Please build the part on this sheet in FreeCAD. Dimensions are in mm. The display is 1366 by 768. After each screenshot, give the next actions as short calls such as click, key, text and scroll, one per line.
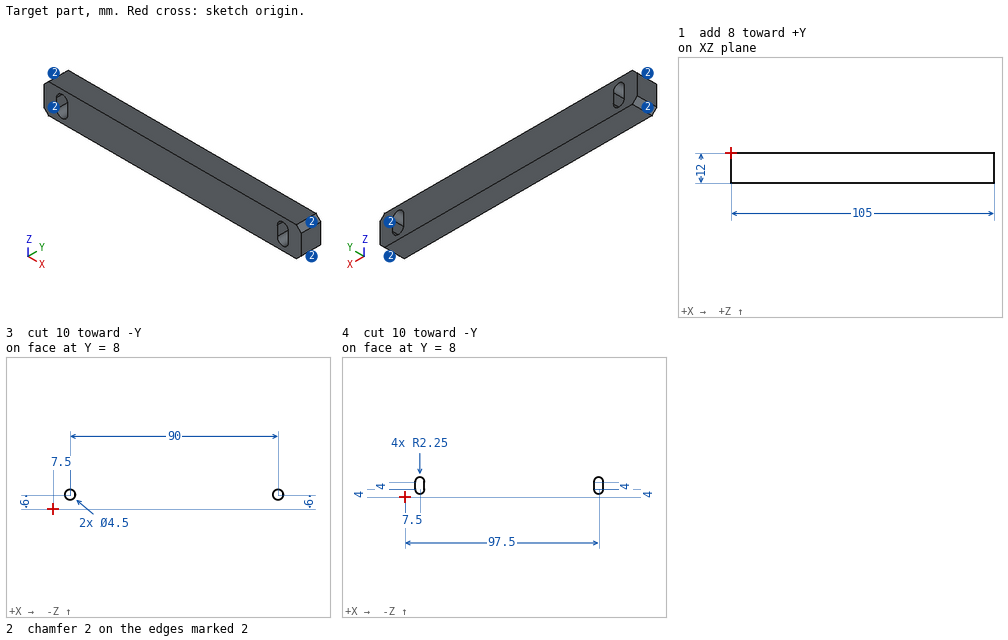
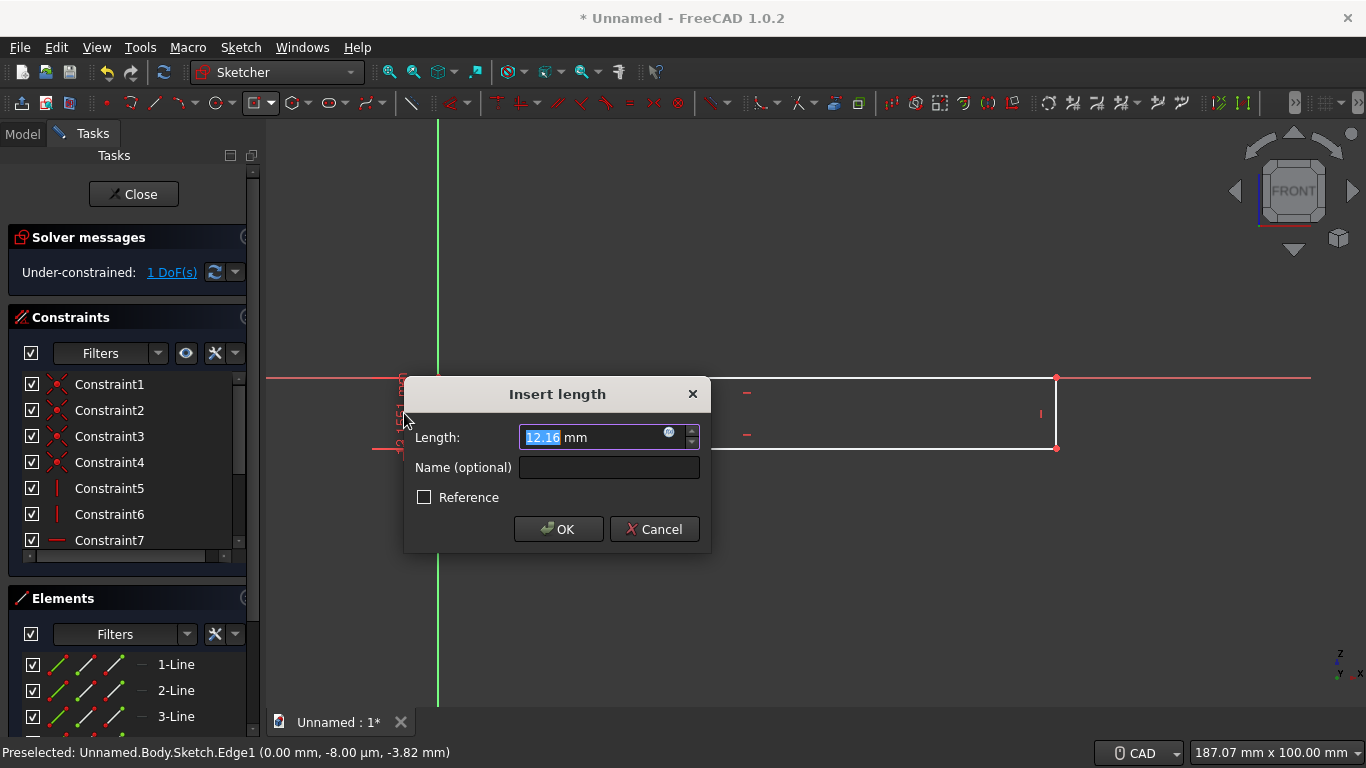
text(12)
key(Return)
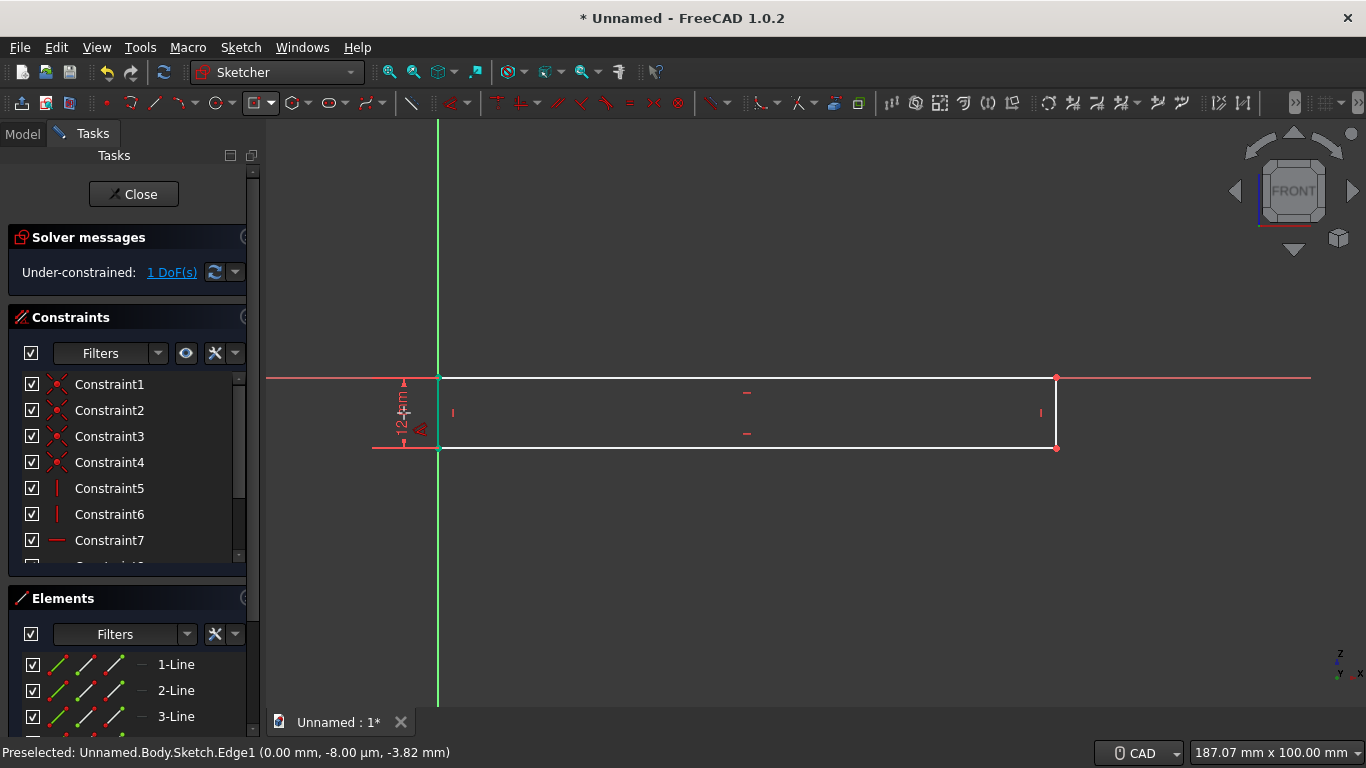
click(624, 448)
click(747, 482)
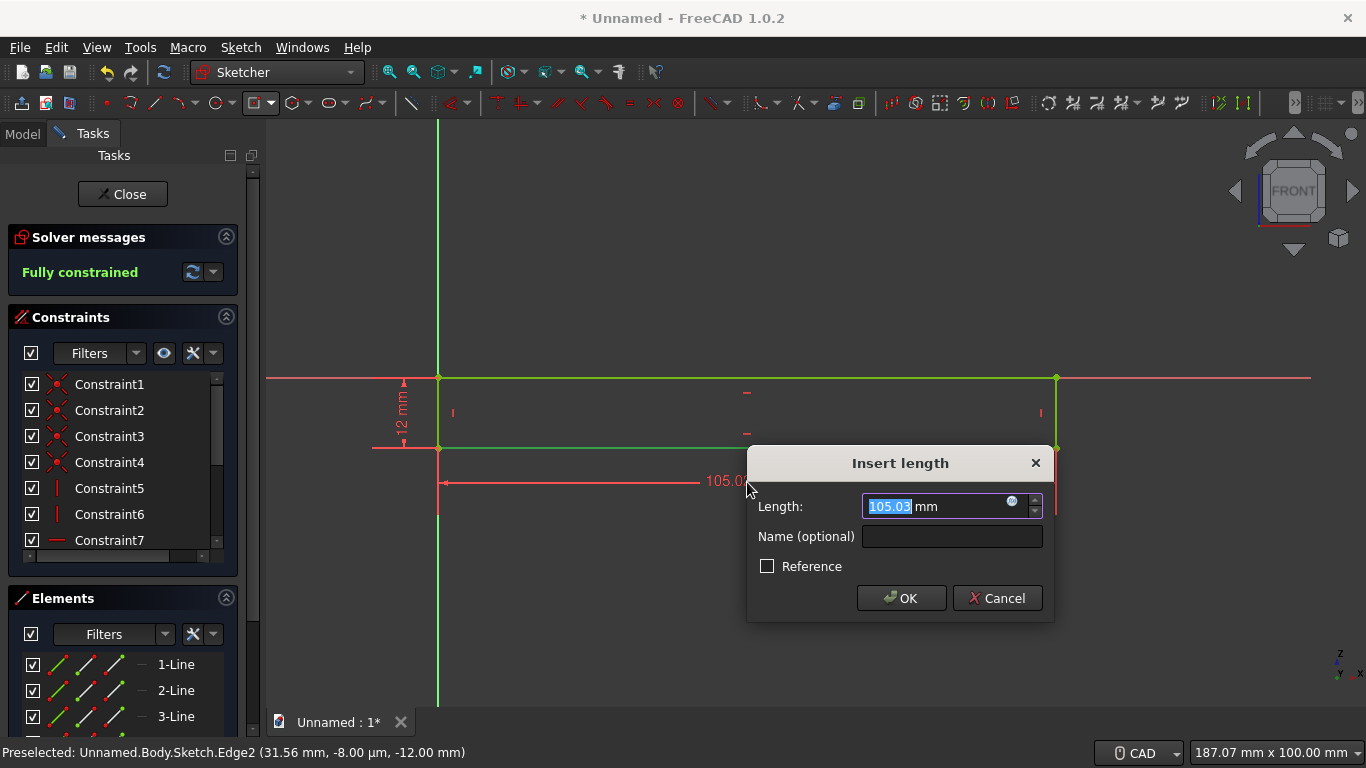
text(105)
key(Return)
key(Escape)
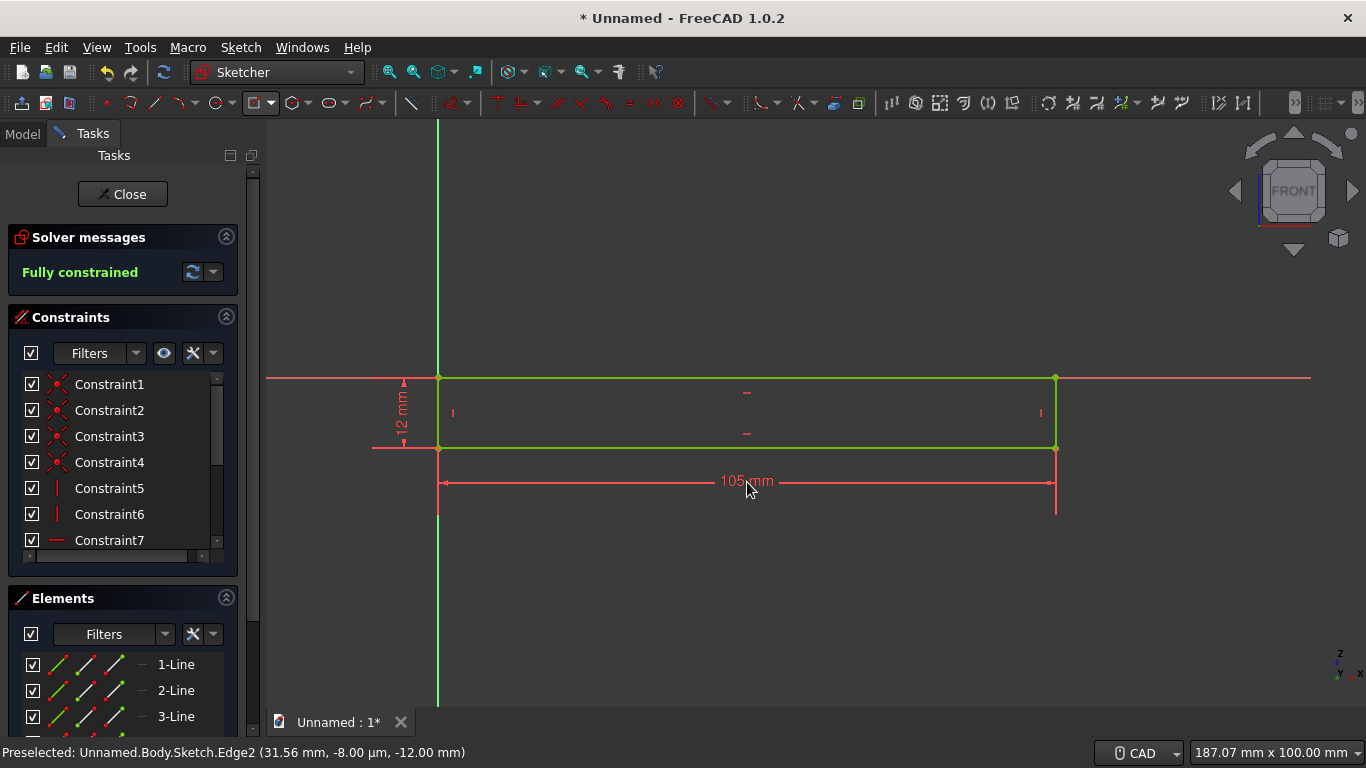
click(123, 194)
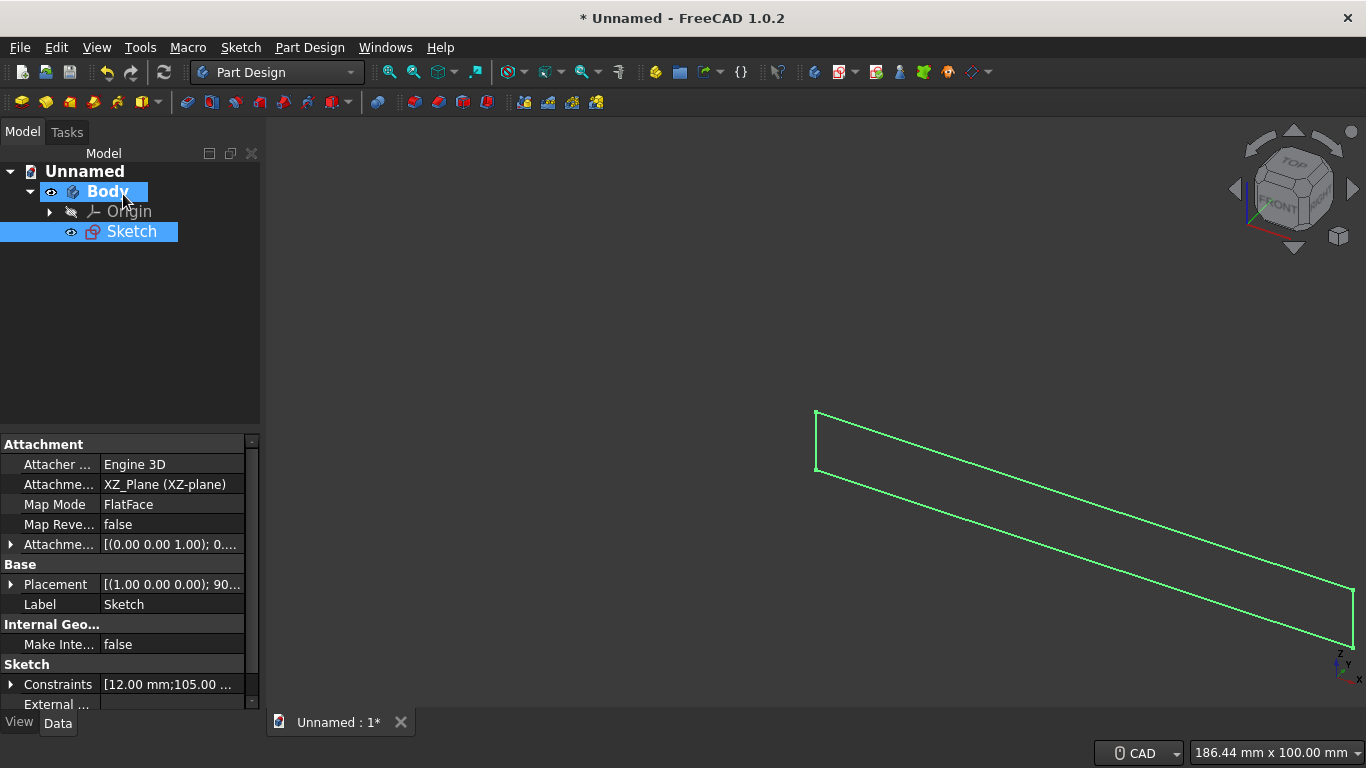
click(22, 102)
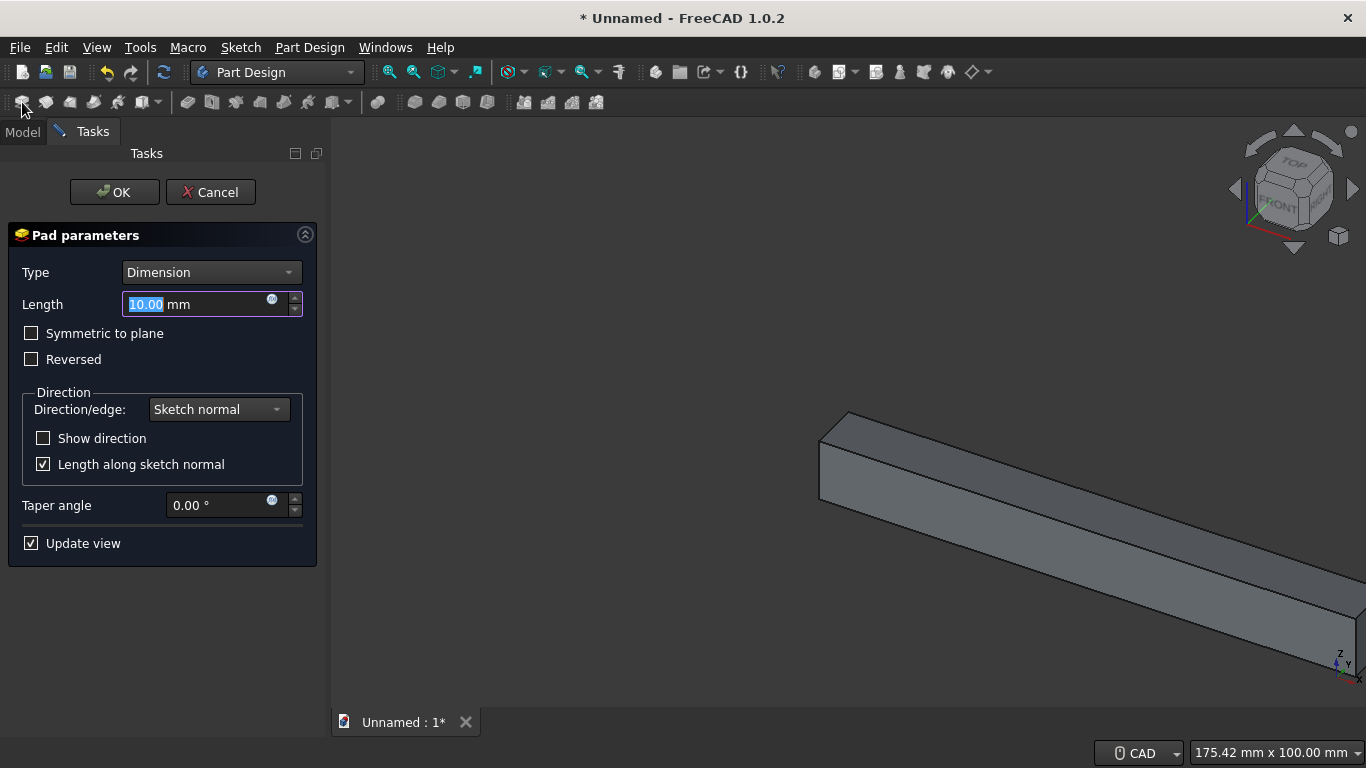
text(8)
key(Tab)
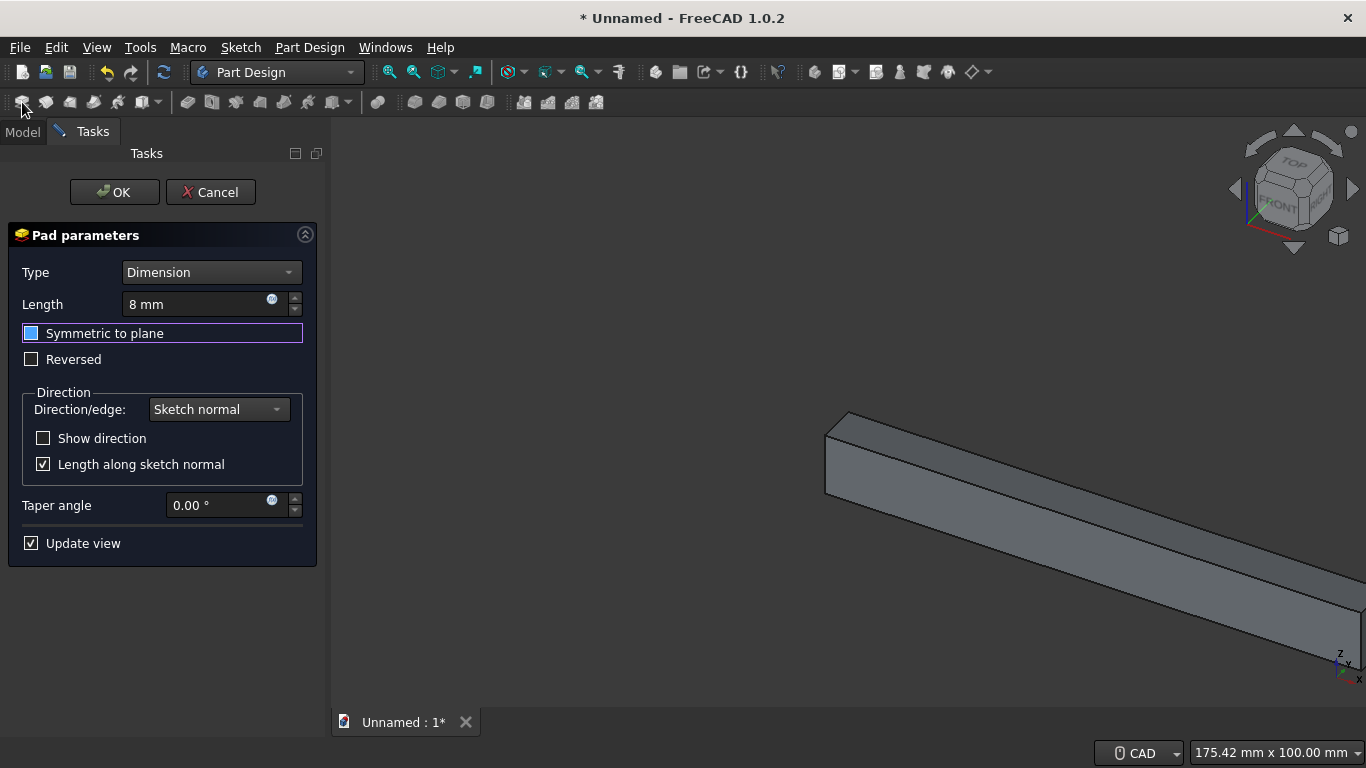
click(30, 359)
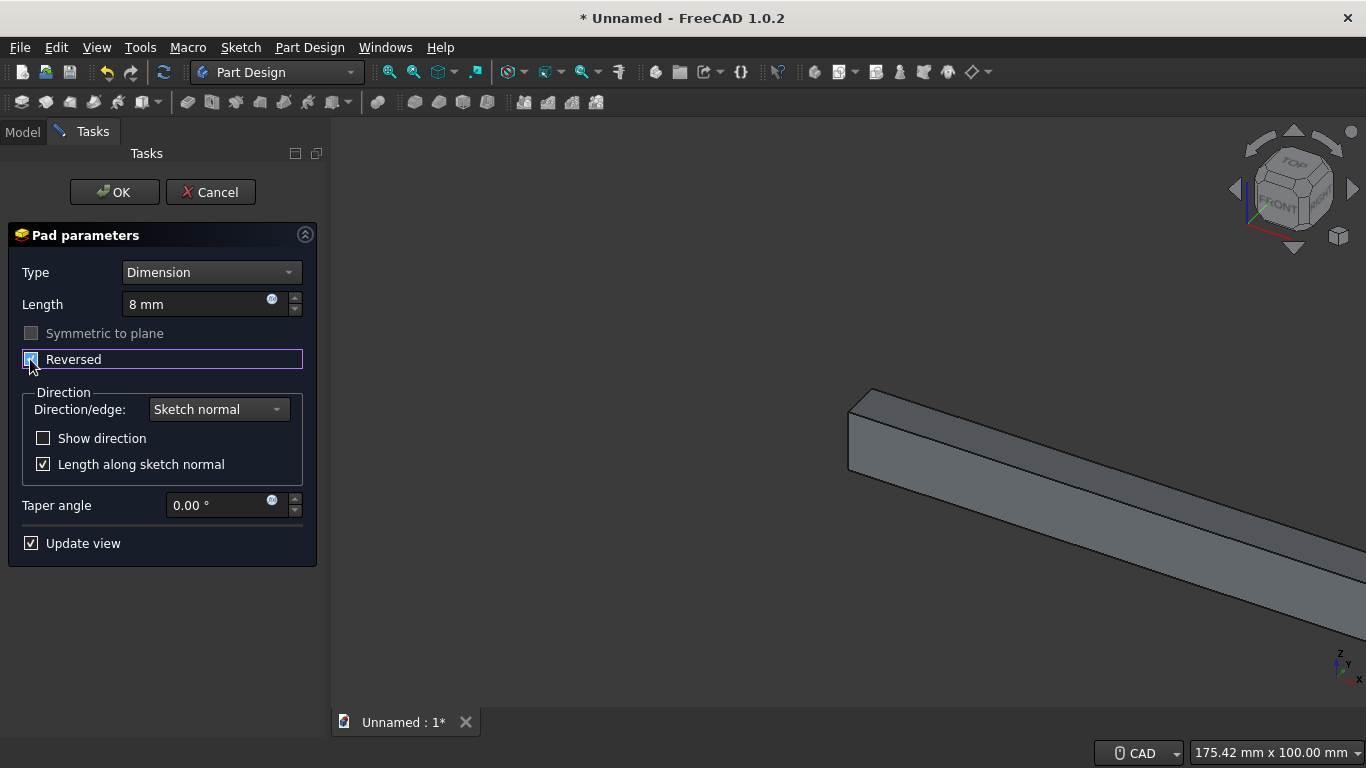
click(115, 192)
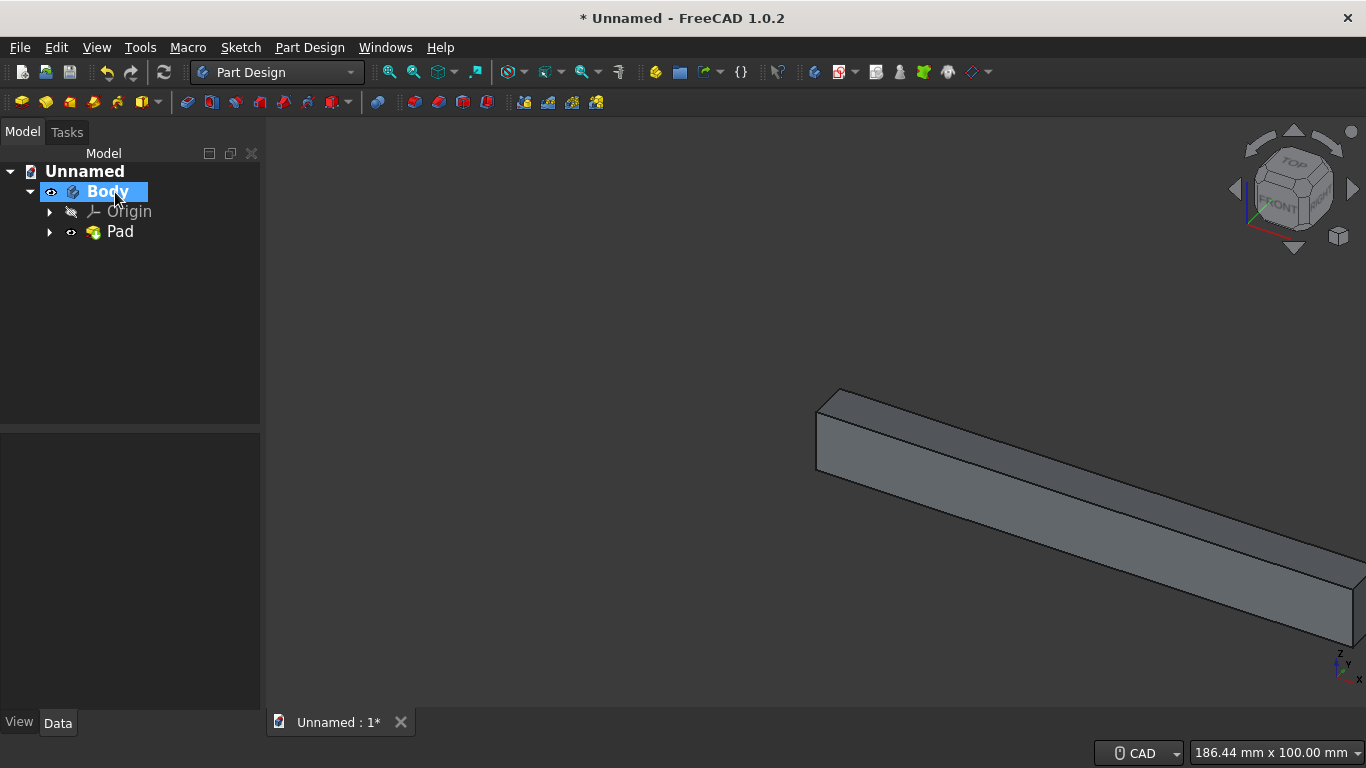
click(390, 72)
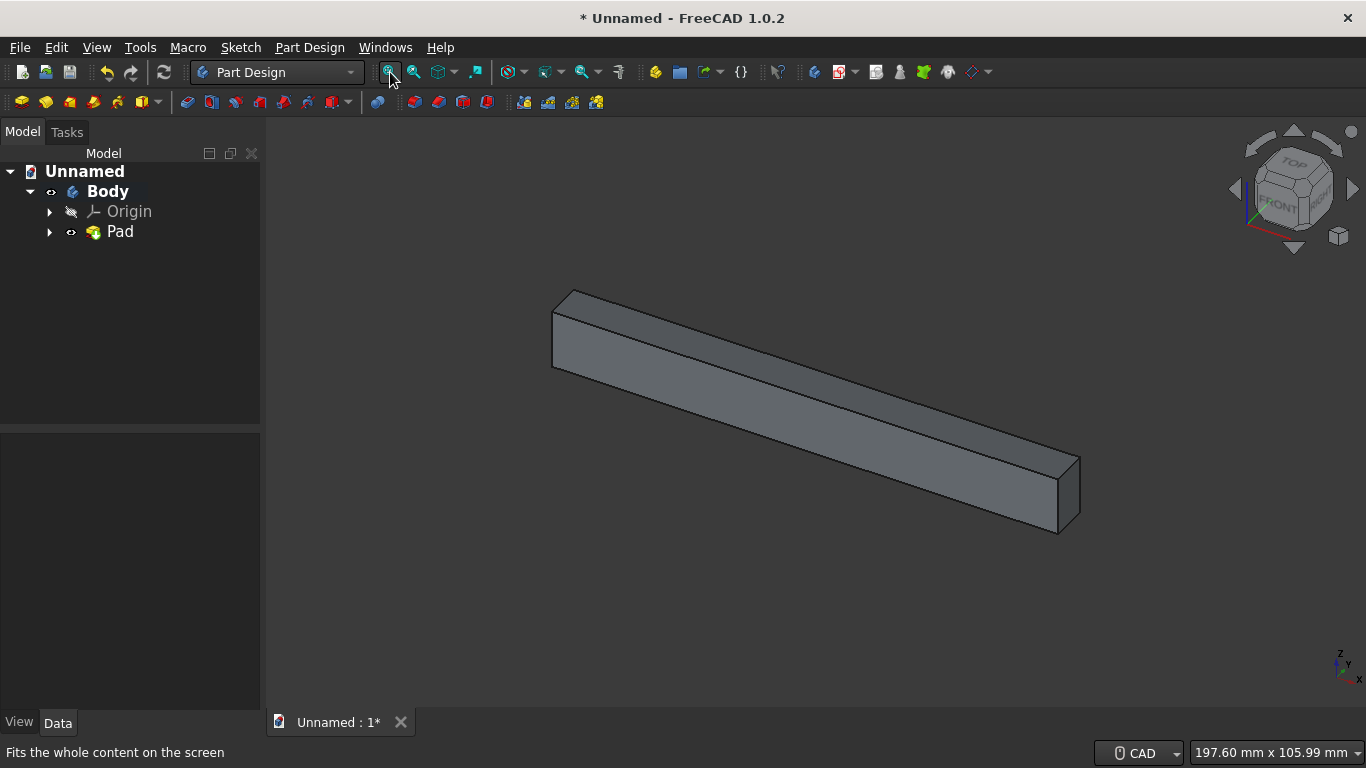
click(1069, 467)